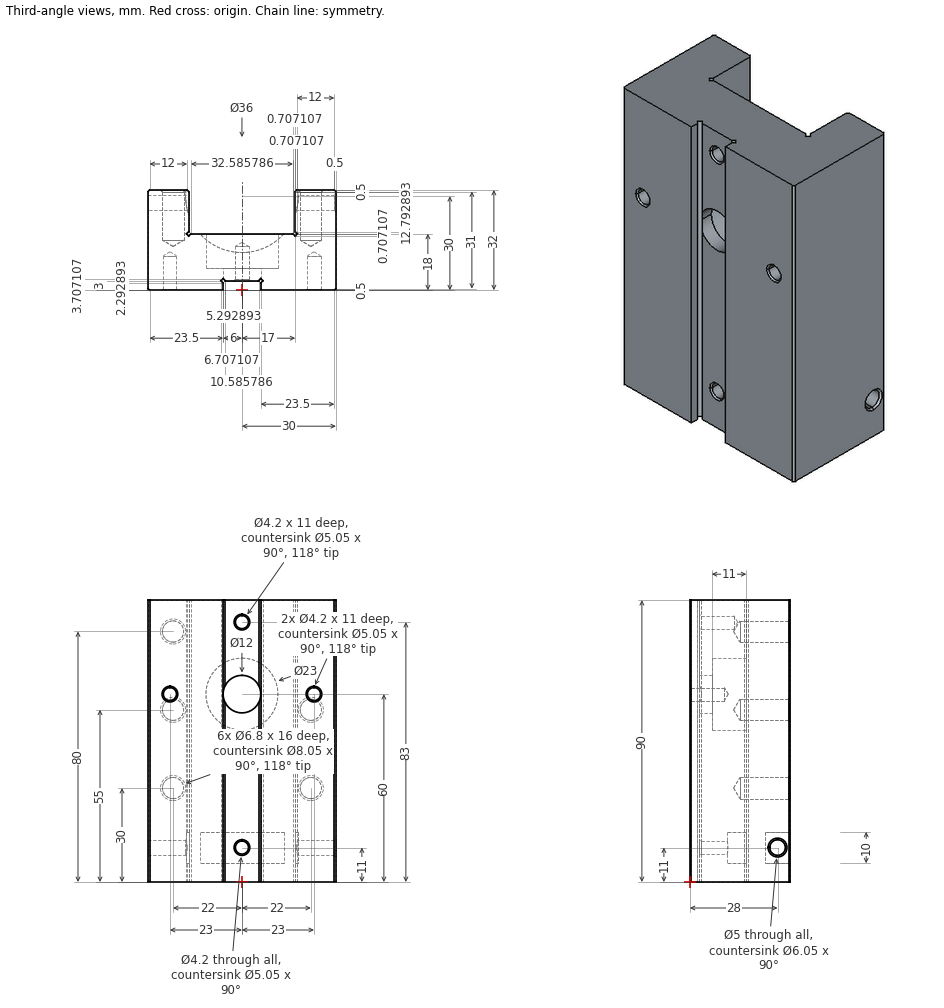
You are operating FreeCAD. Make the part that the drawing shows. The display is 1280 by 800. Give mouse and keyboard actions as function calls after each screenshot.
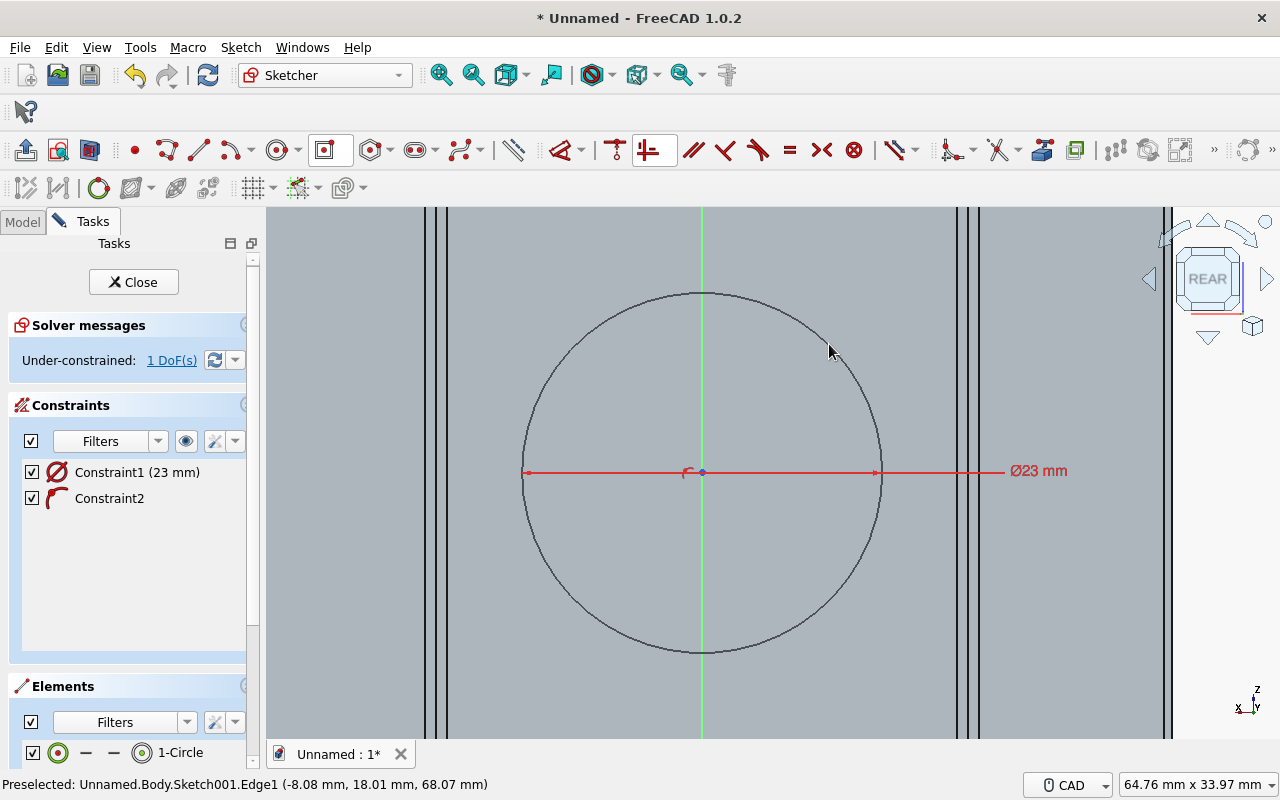
click(560, 150)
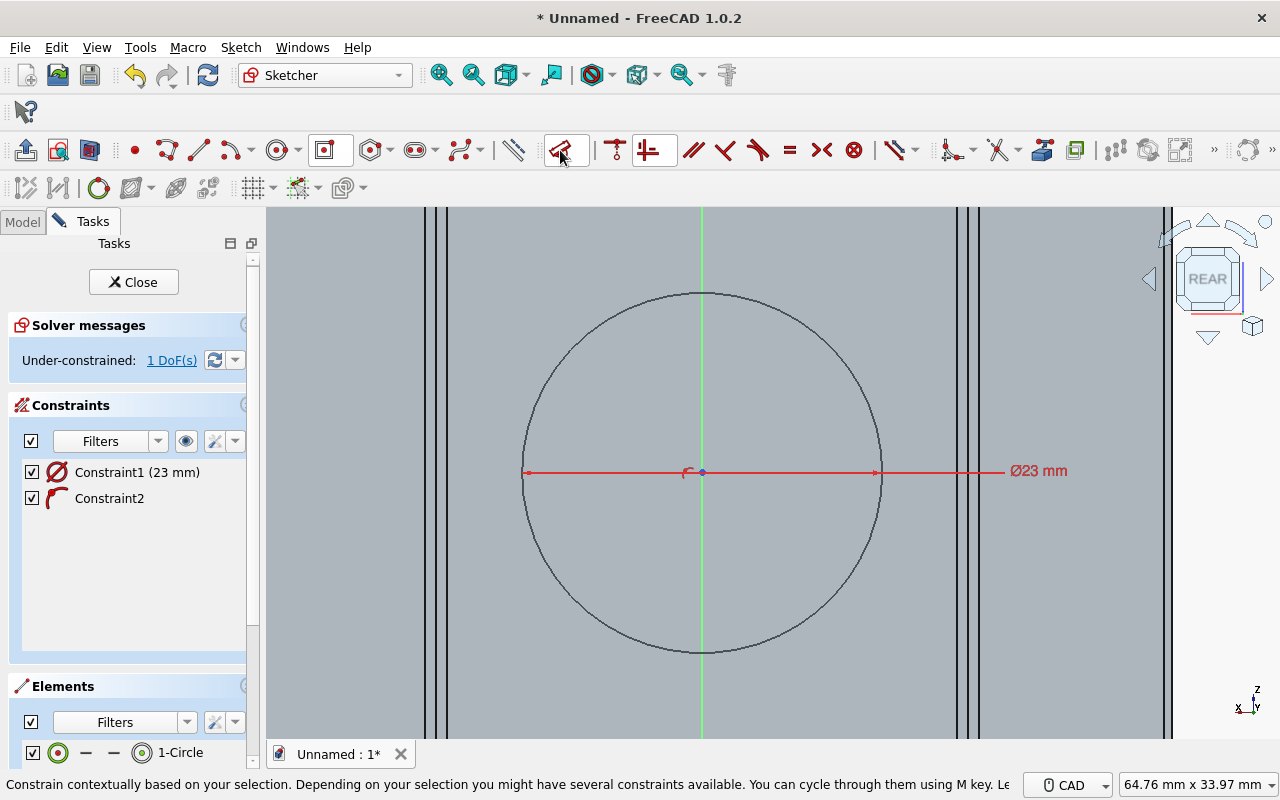
click(702, 473)
click(736, 592)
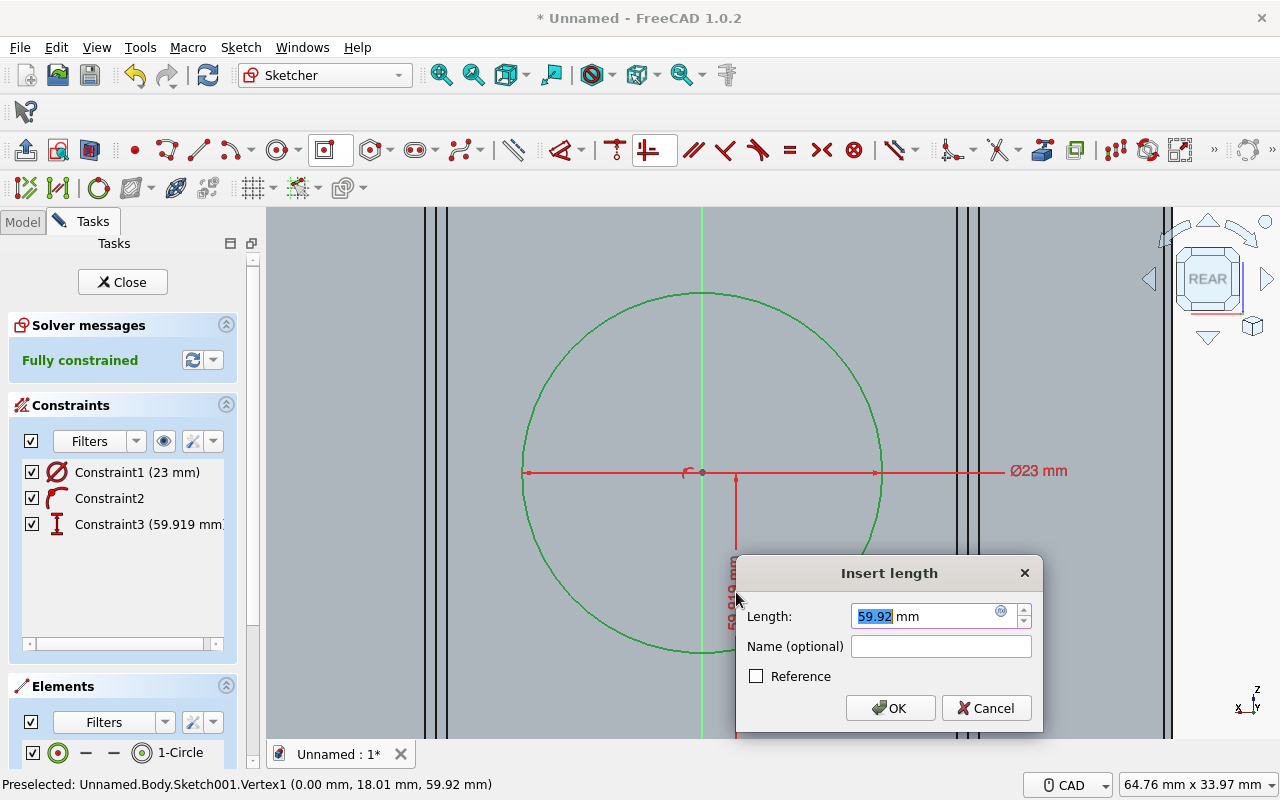
text(60)
key(Return)
key(Escape)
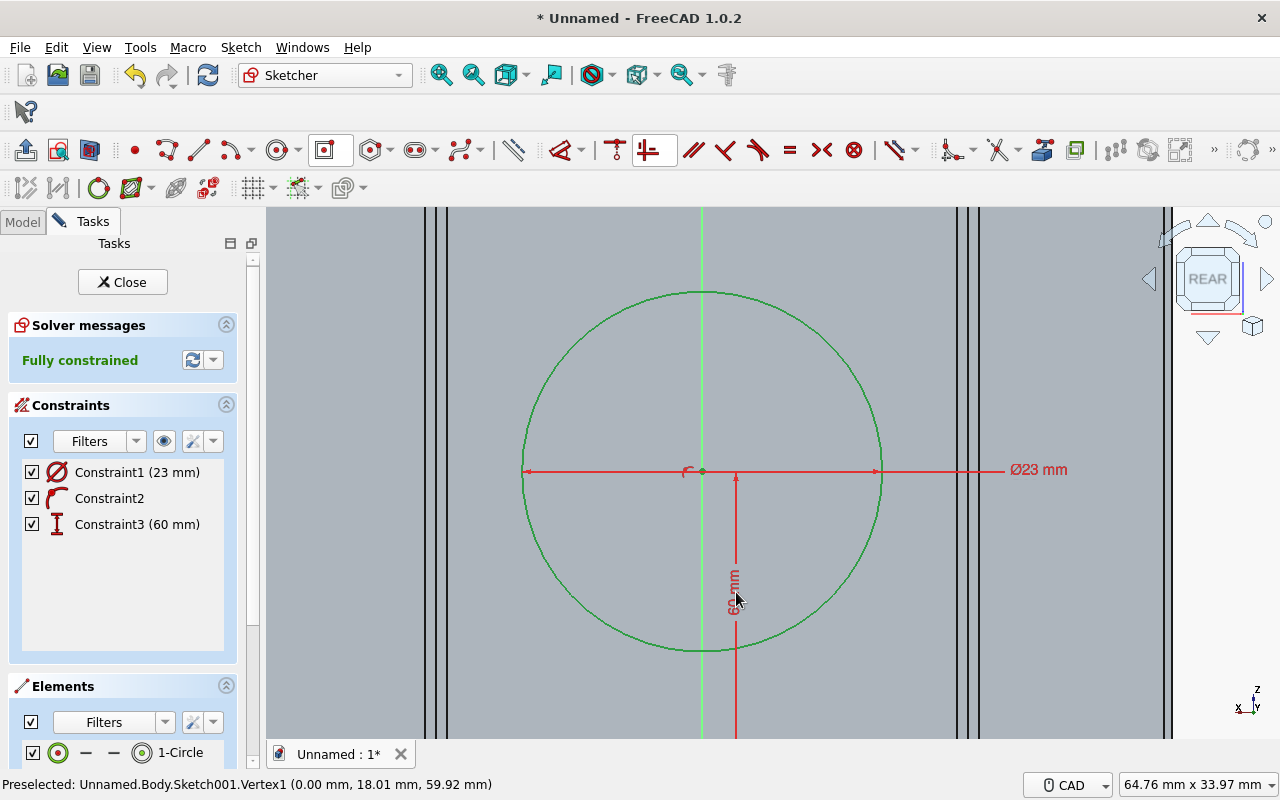
click(123, 282)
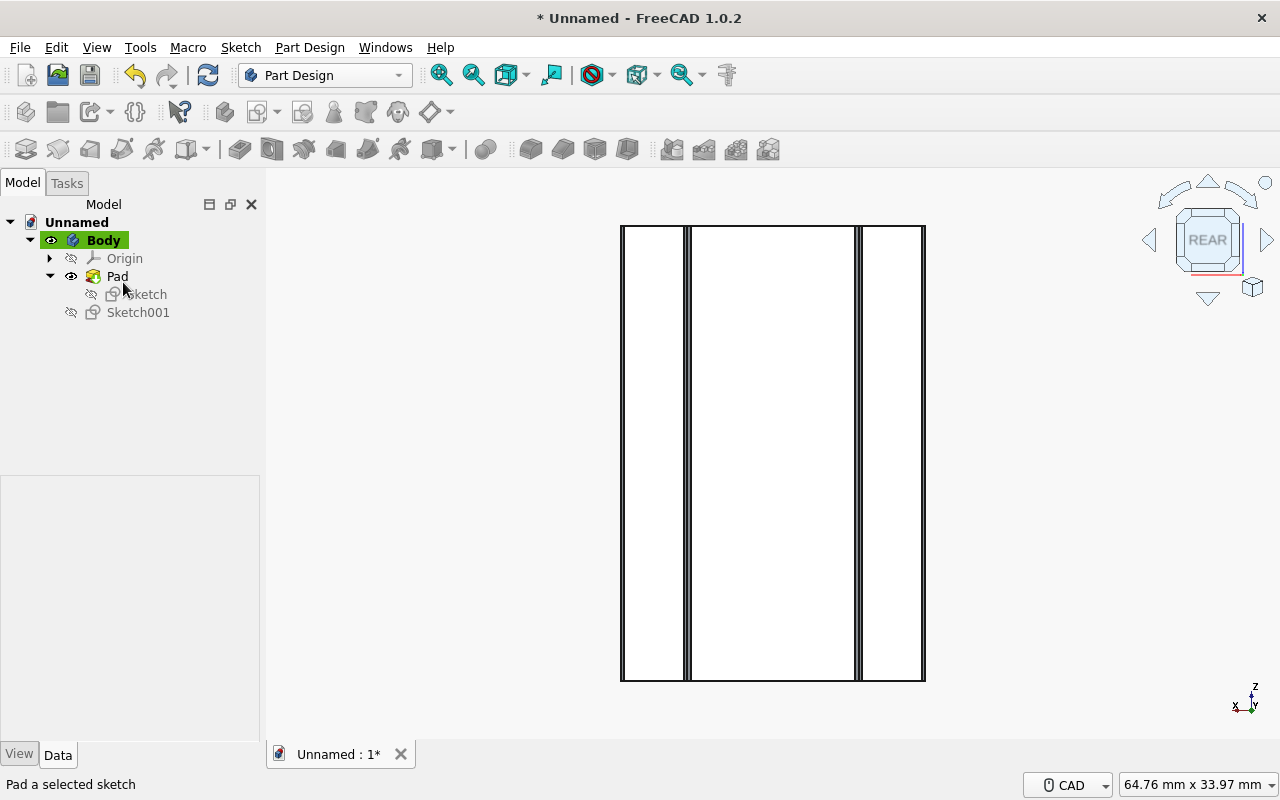
click(240, 150)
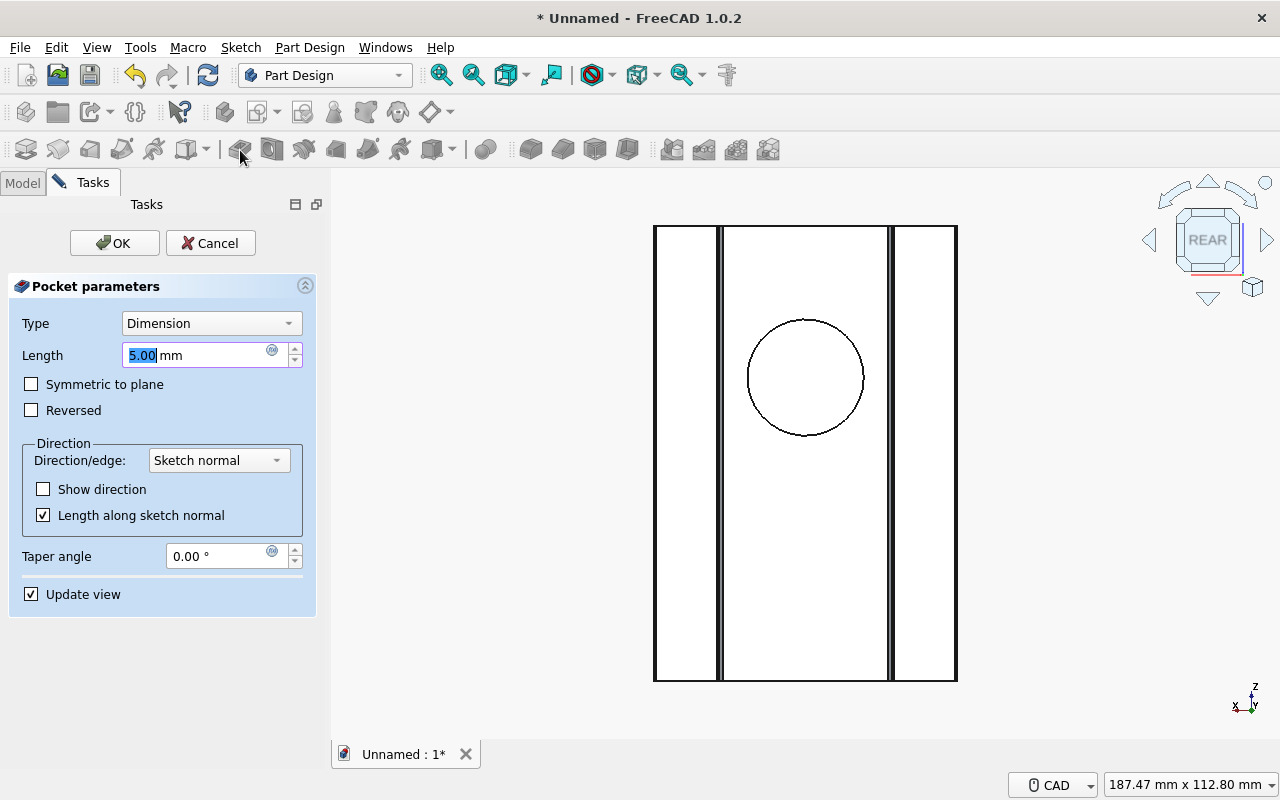
text(11)
key(Tab)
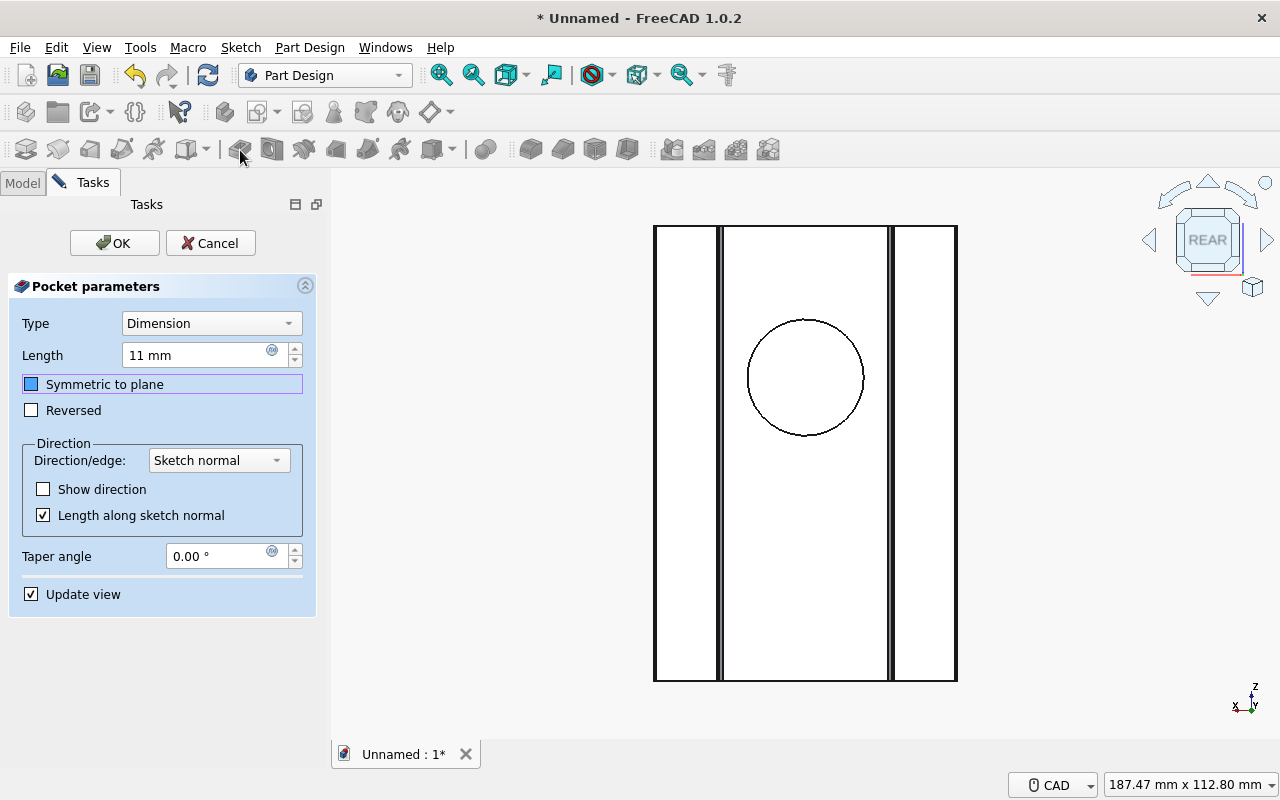
click(115, 243)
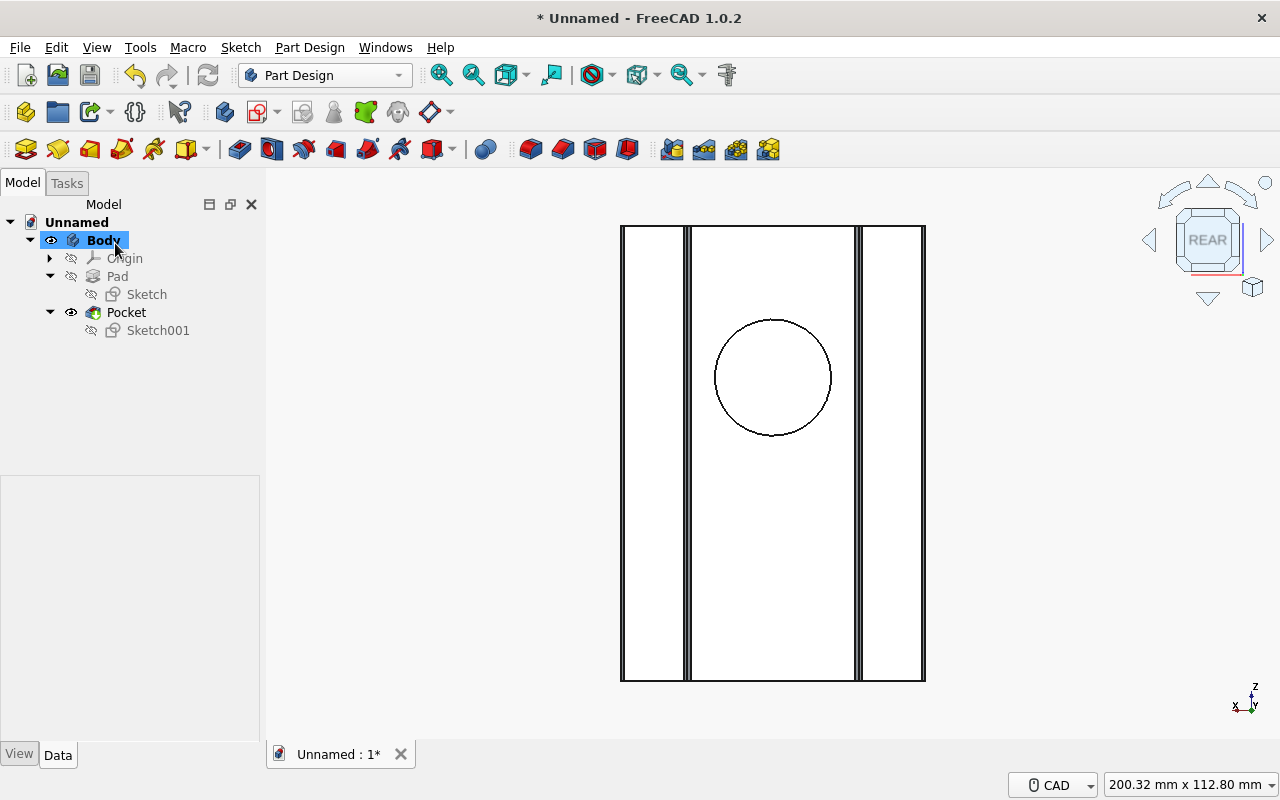
click(773, 377)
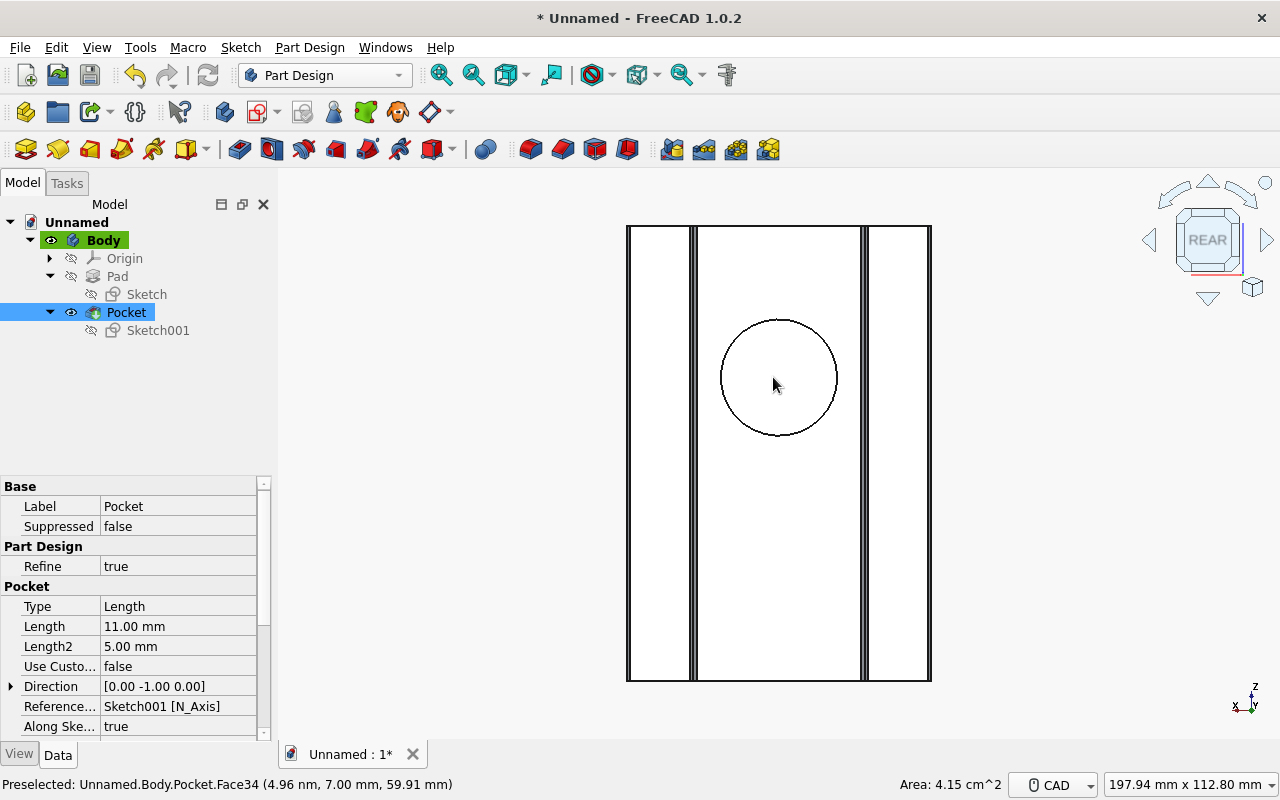
click(258, 112)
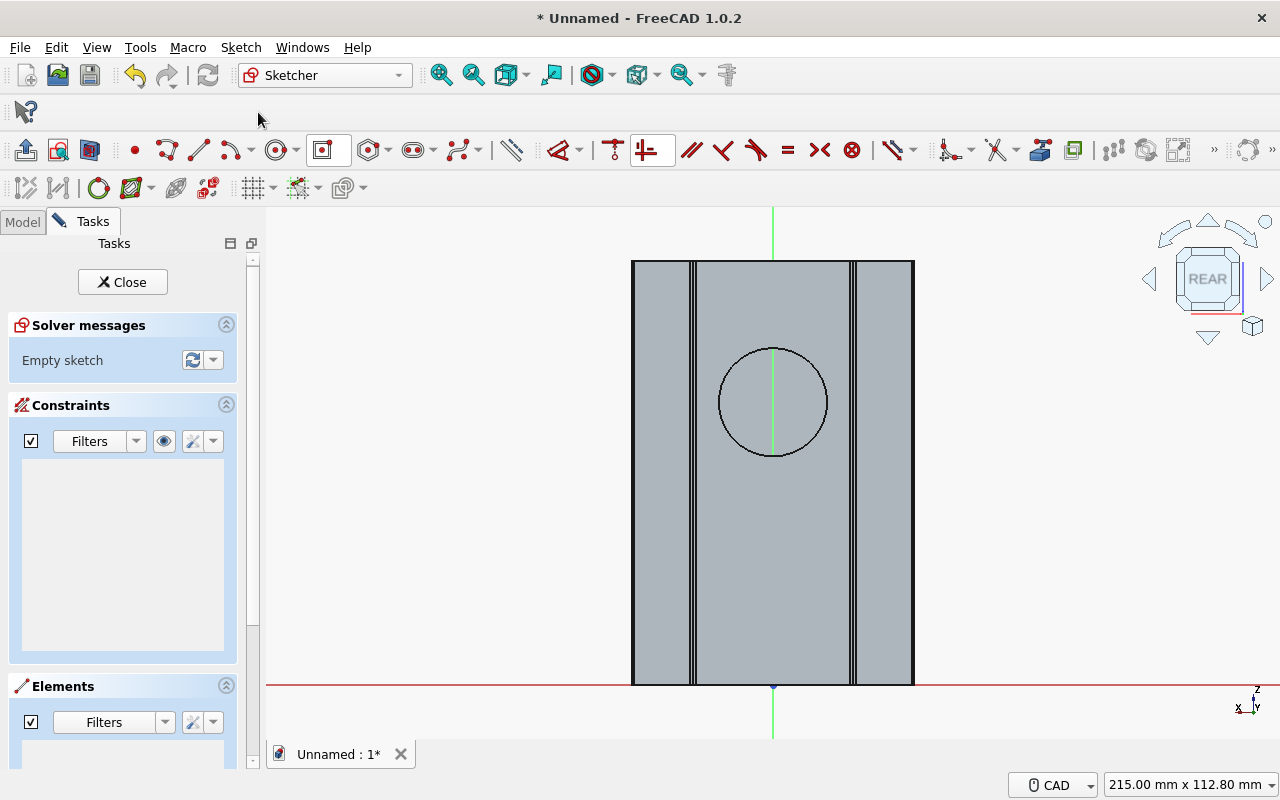
click(90, 150)